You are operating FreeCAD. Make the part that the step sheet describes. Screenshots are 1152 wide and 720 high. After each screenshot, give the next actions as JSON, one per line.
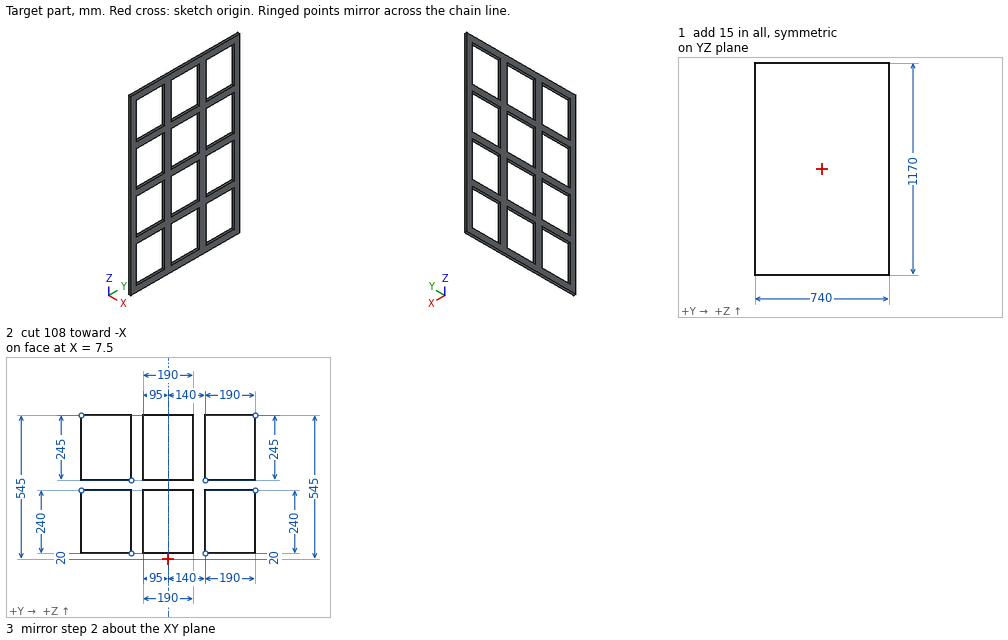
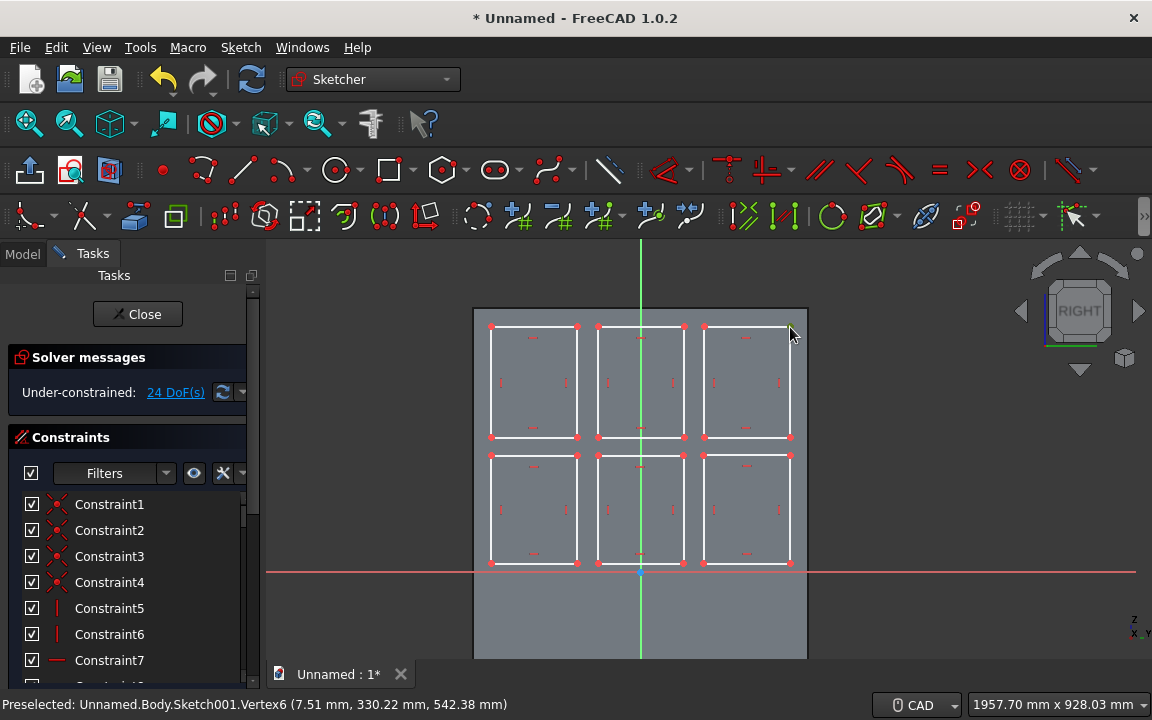
{"action": "left_click", "coordinate": [491, 327]}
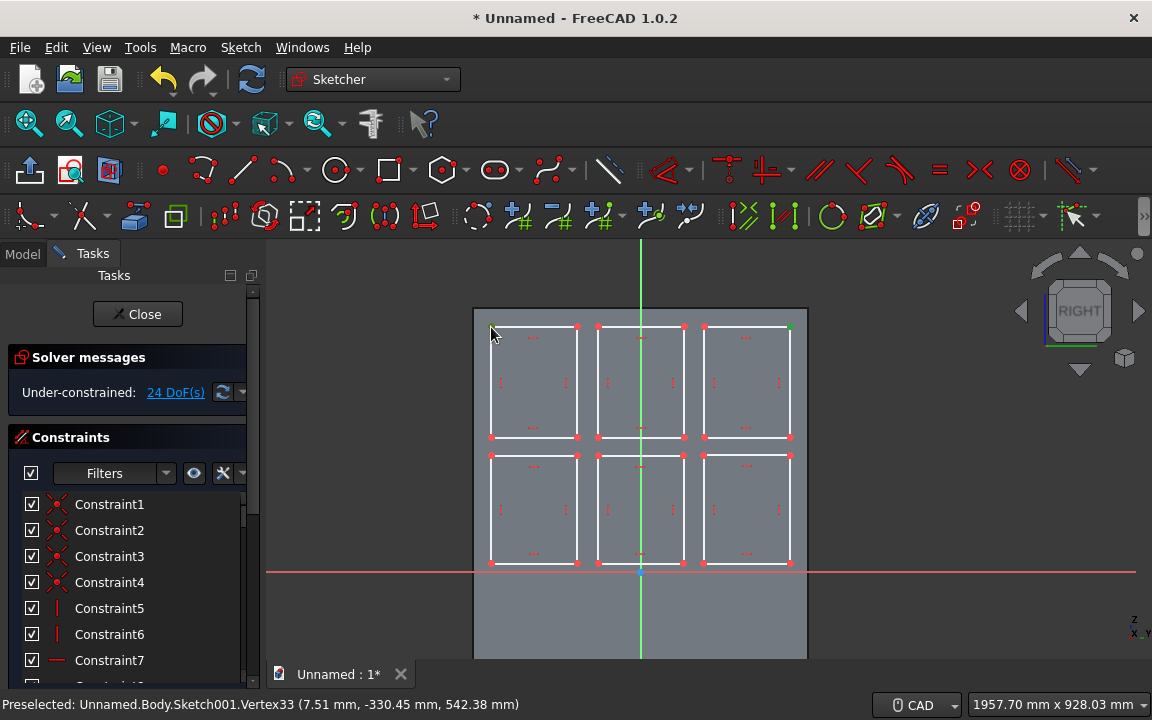
{"action": "left_click", "coordinate": [641, 605]}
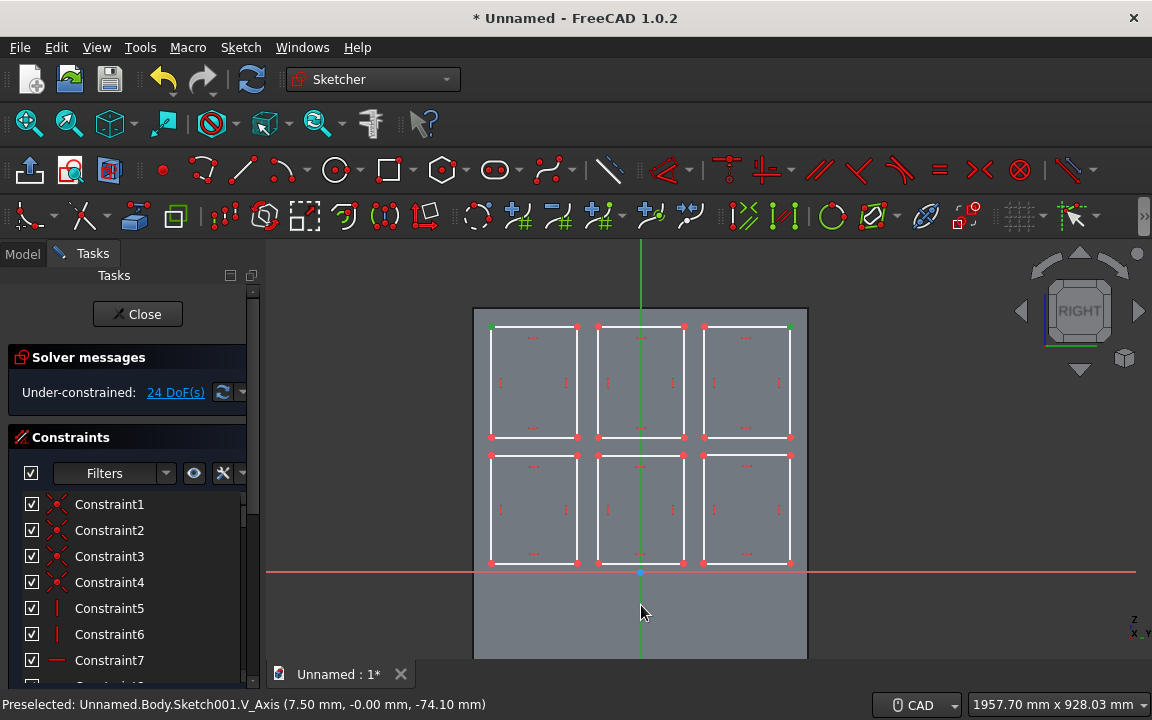
{"action": "key", "text": "s"}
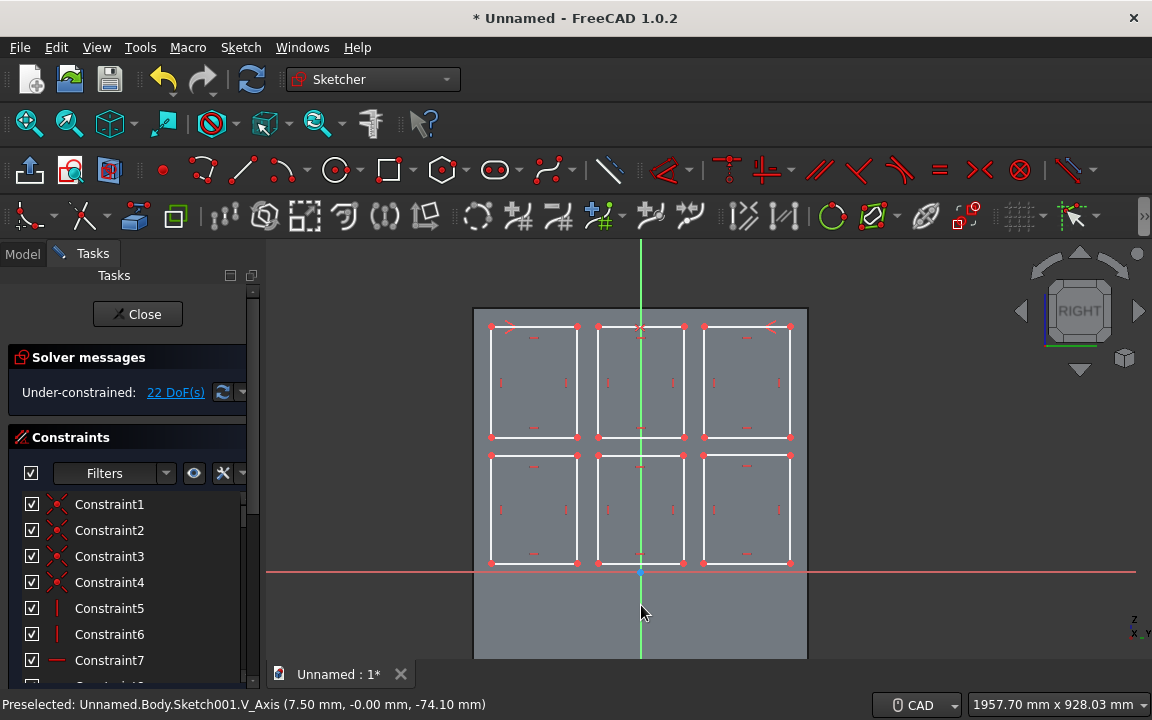
{"action": "left_click", "coordinate": [704, 438]}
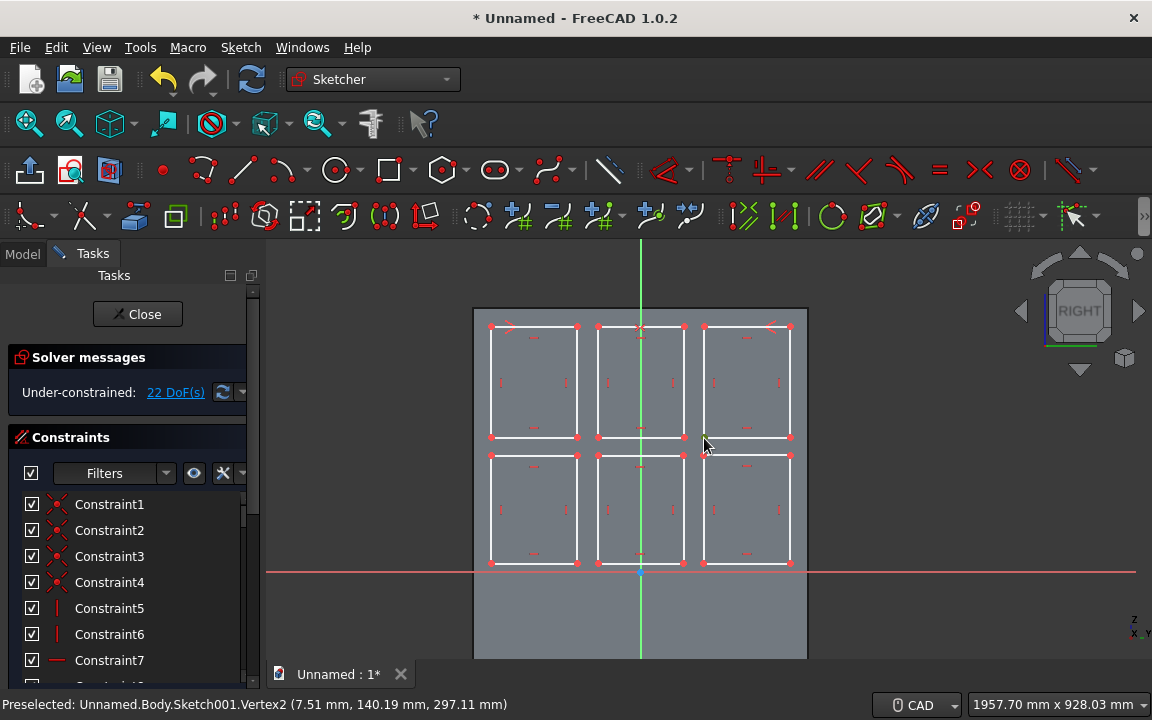
{"action": "left_click", "coordinate": [577, 438]}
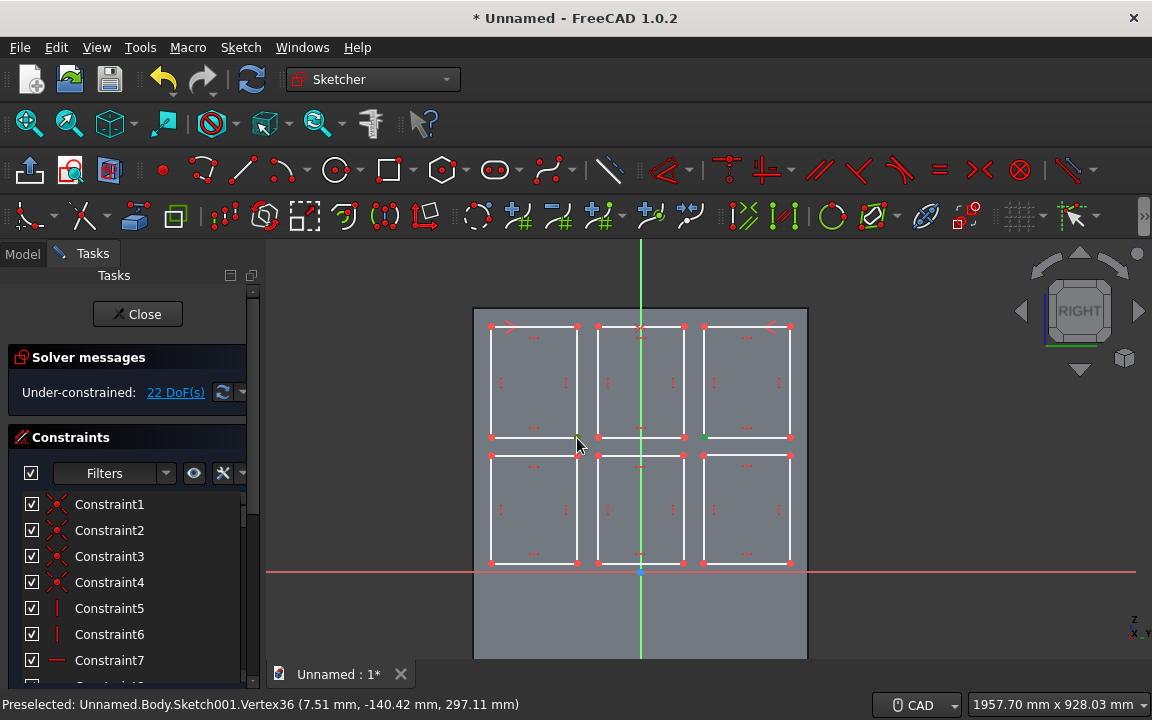
{"action": "left_click", "coordinate": [641, 605]}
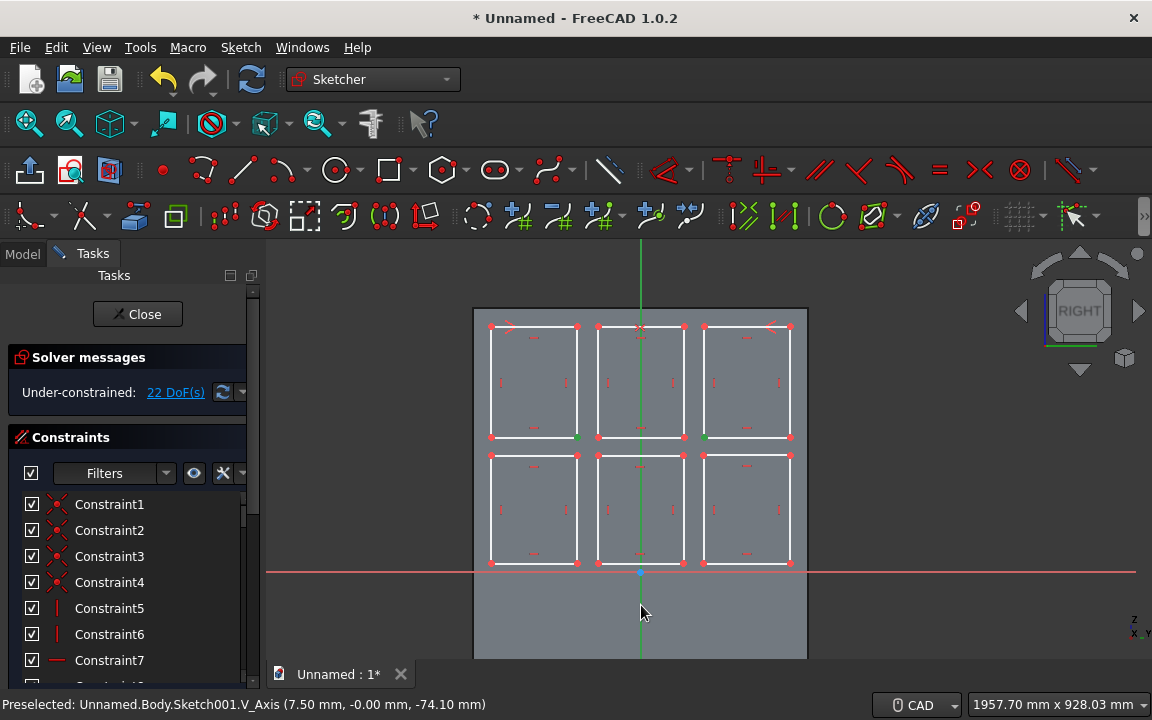
{"action": "key", "text": "s"}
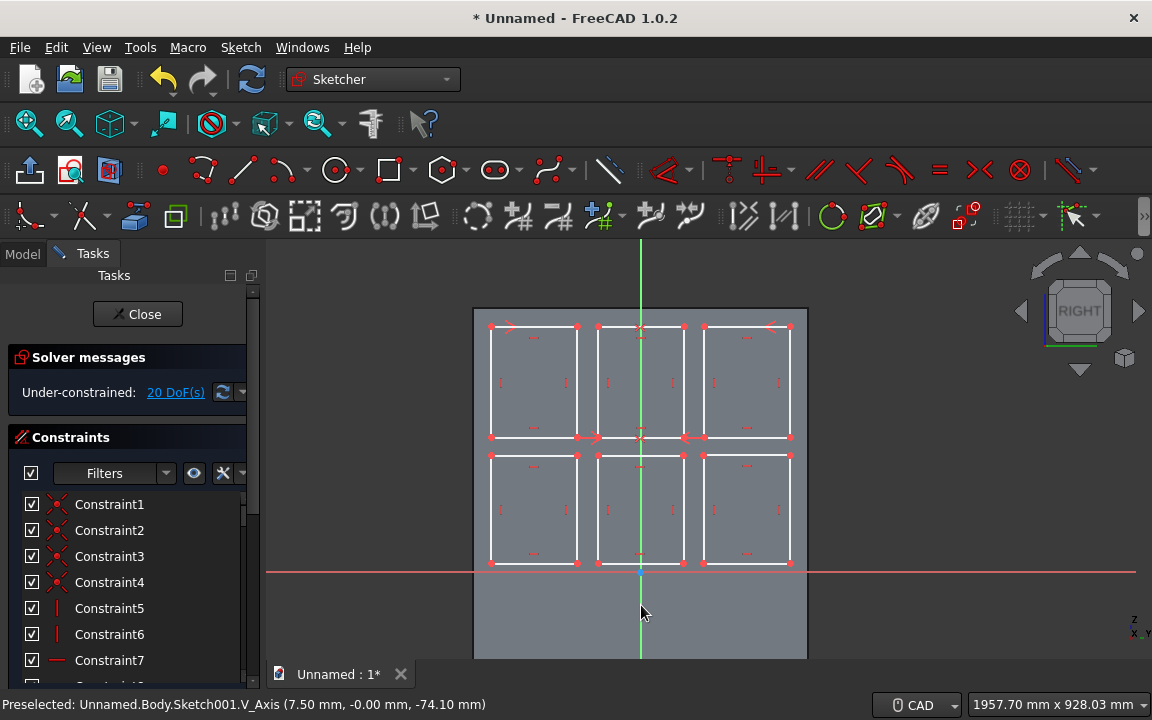
{"action": "left_click", "coordinate": [790, 455]}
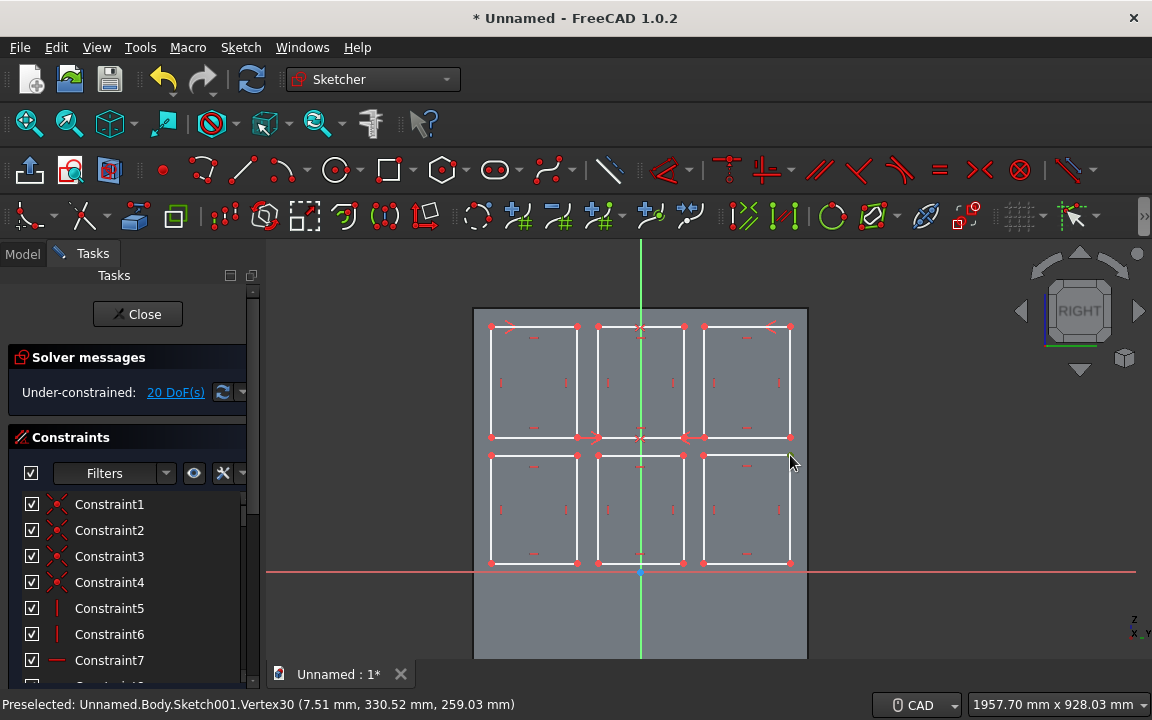
{"action": "left_click", "coordinate": [491, 456]}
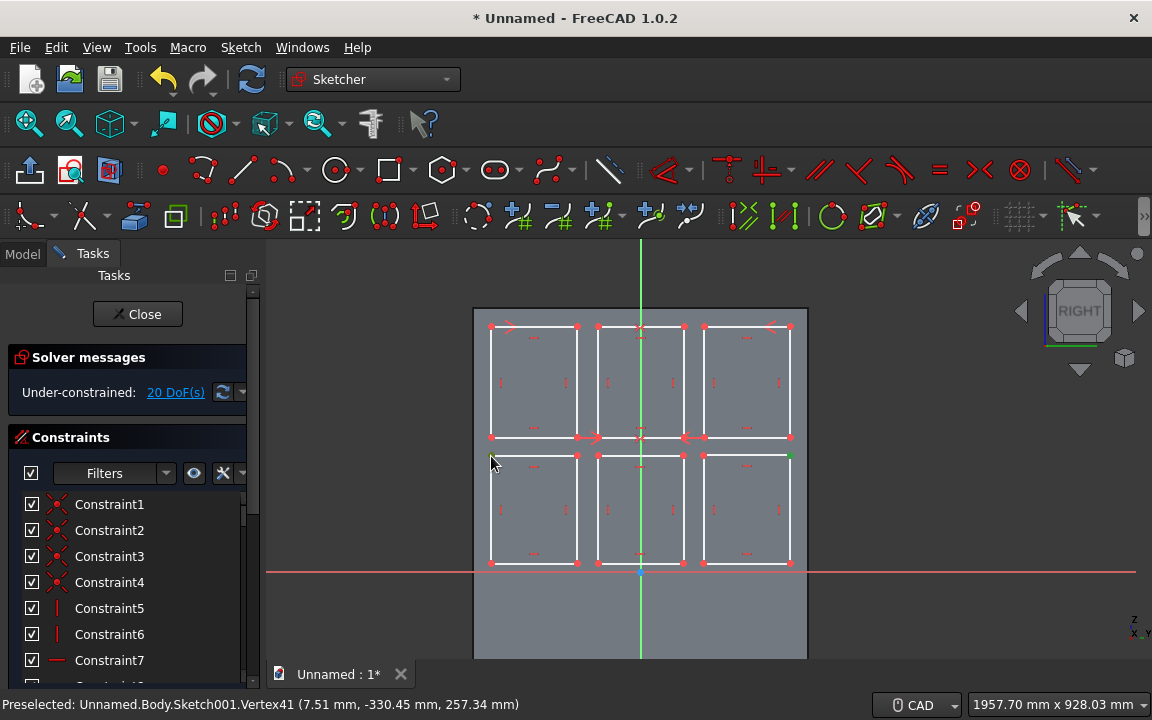
{"action": "left_click", "coordinate": [641, 605]}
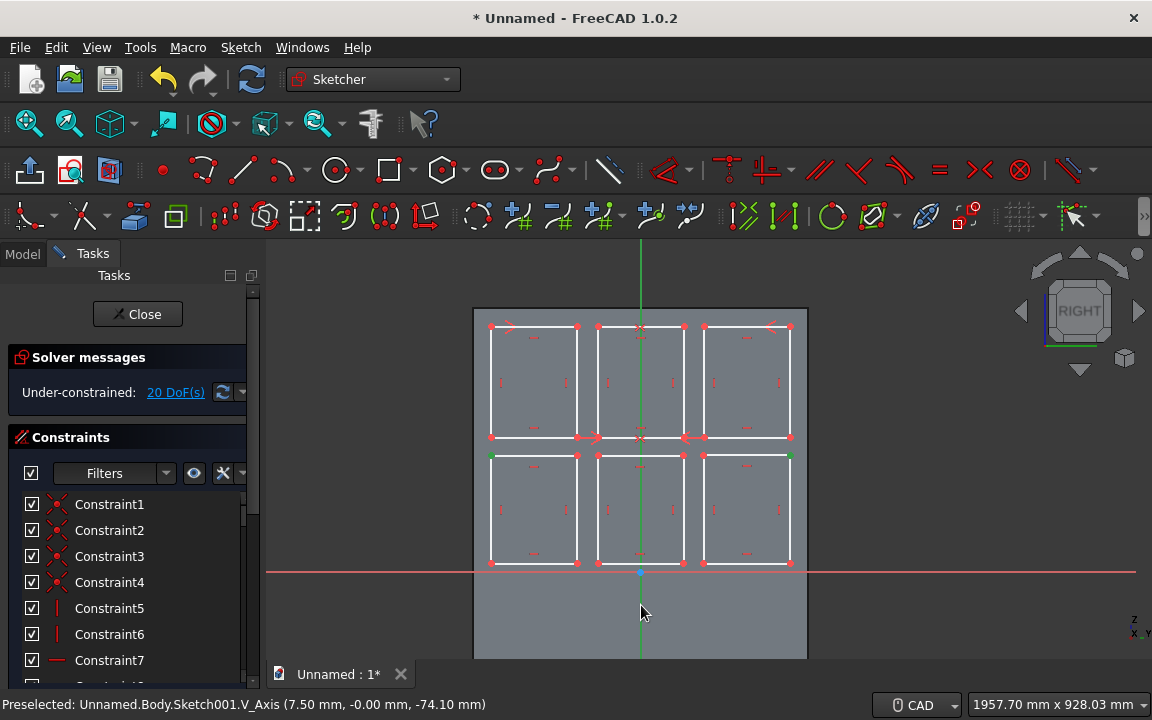
{"action": "key", "text": "s"}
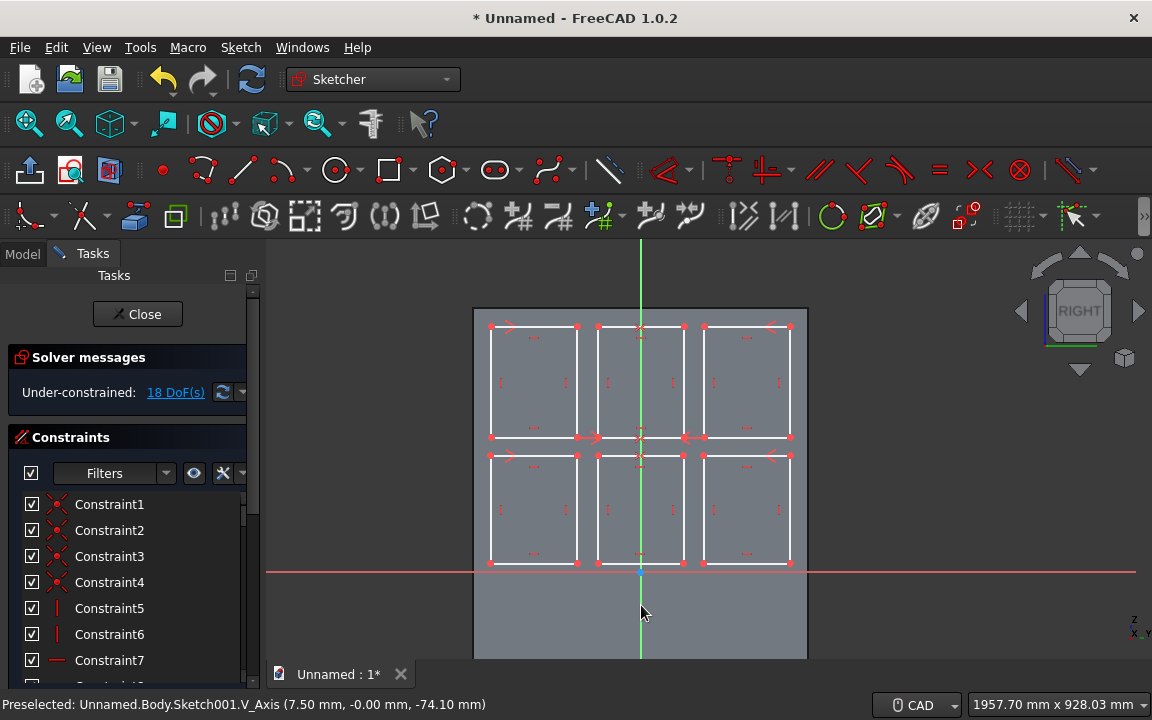
{"action": "left_click", "coordinate": [704, 564]}